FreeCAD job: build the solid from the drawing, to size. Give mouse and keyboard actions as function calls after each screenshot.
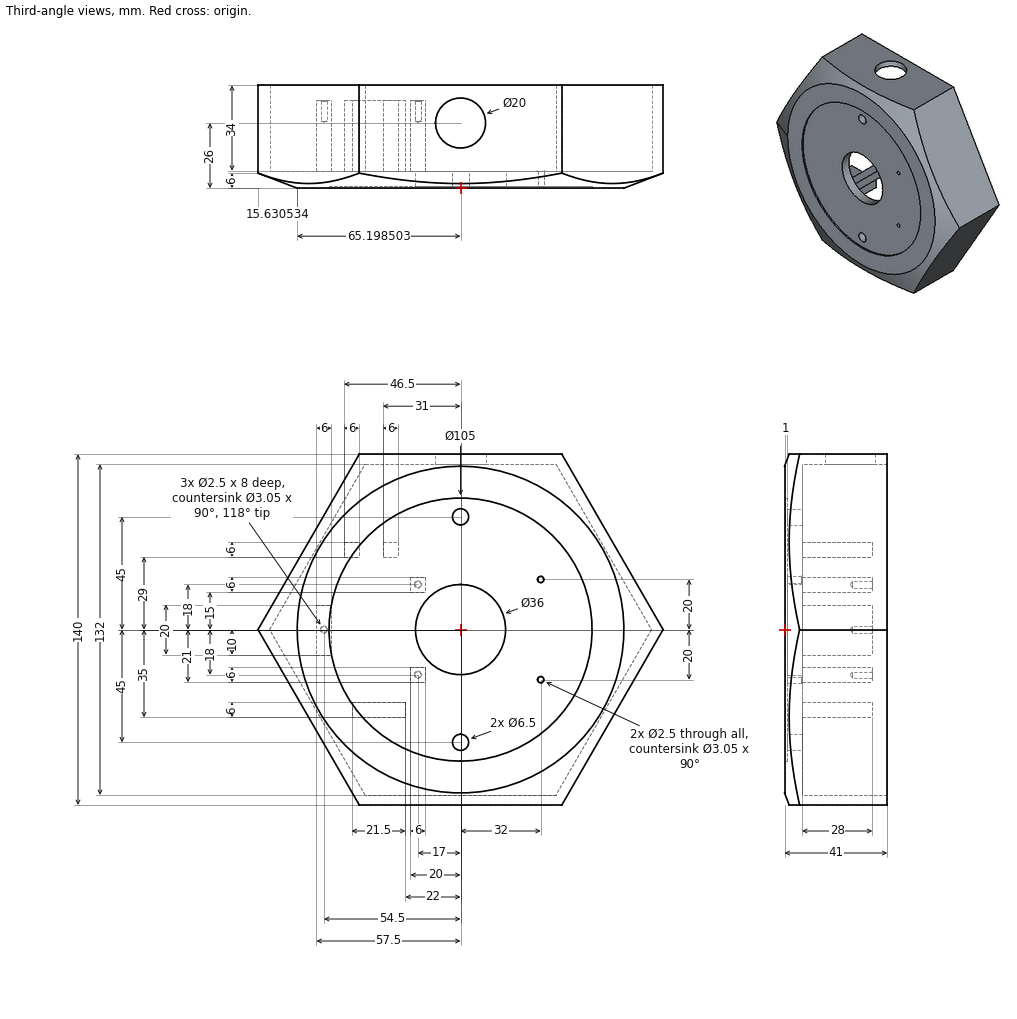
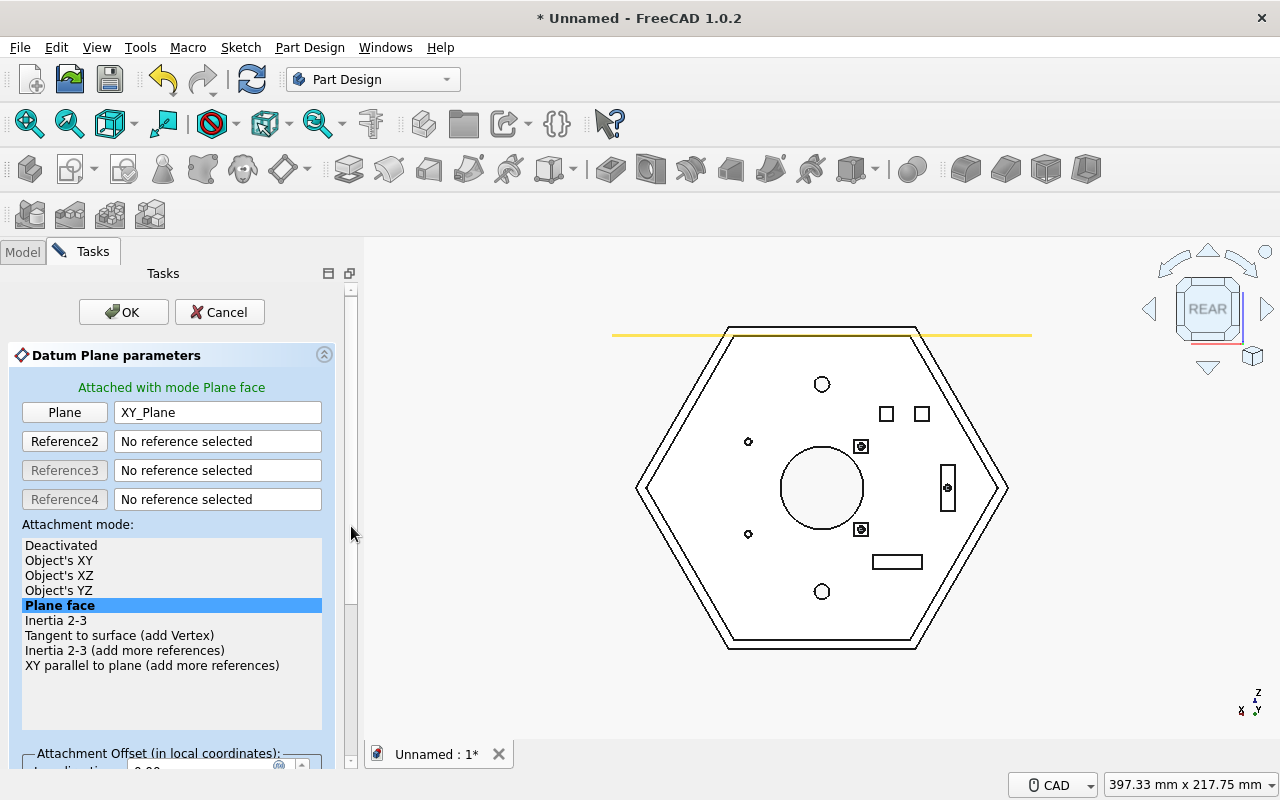
click(124, 312)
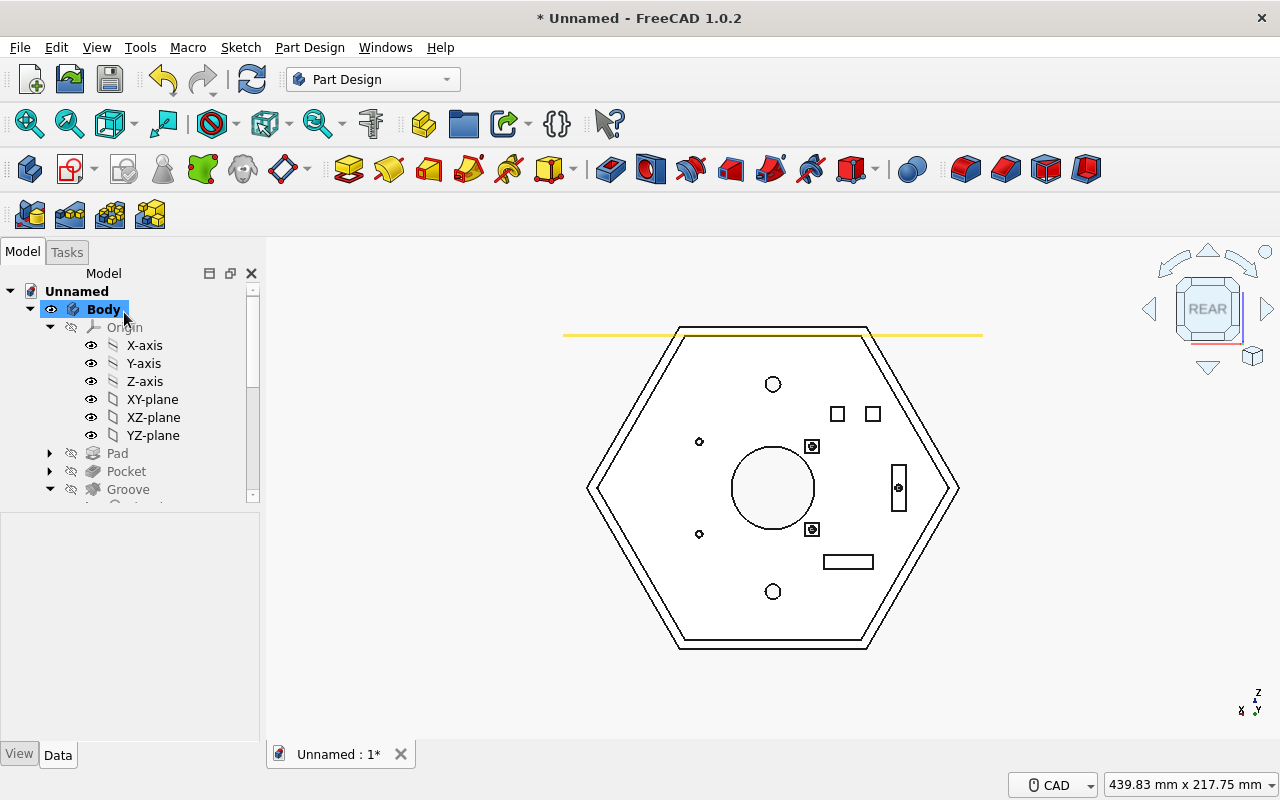
scroll(100, 395, down, 3)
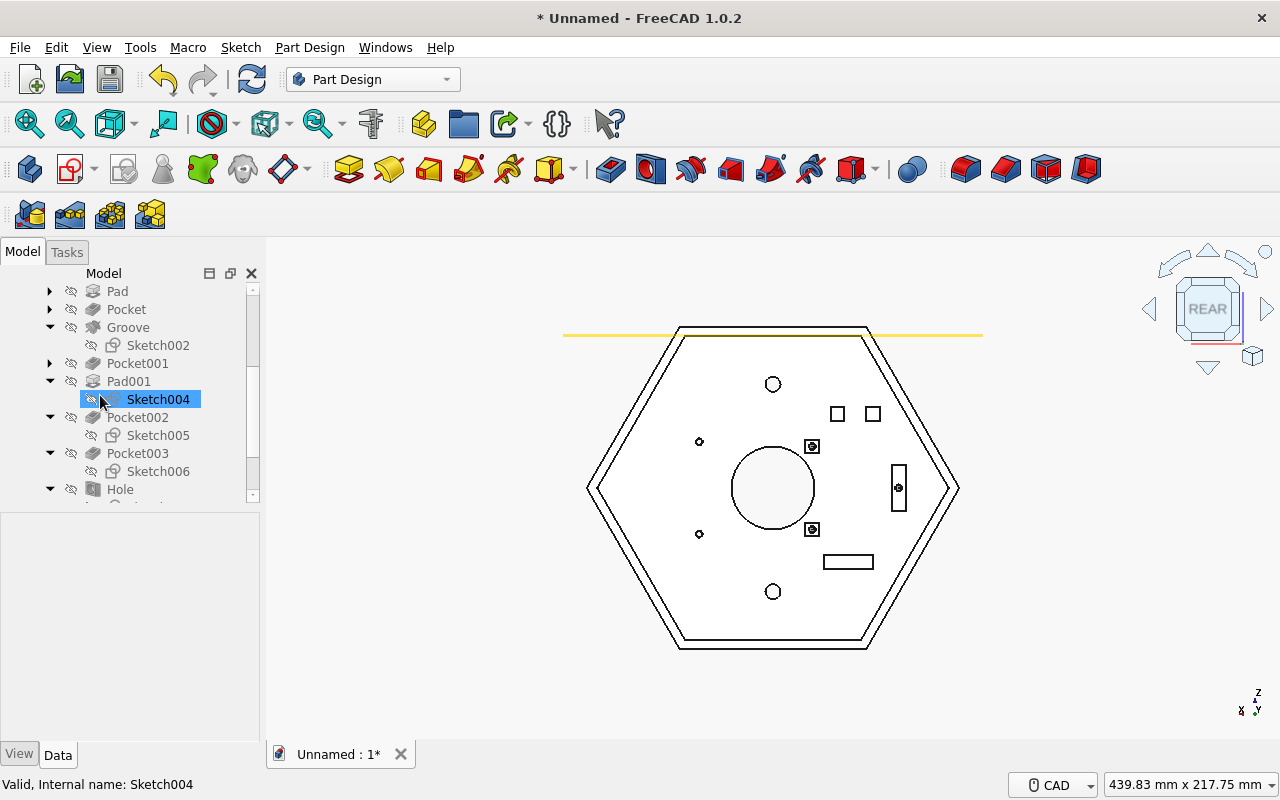
scroll(140, 395, up, 15)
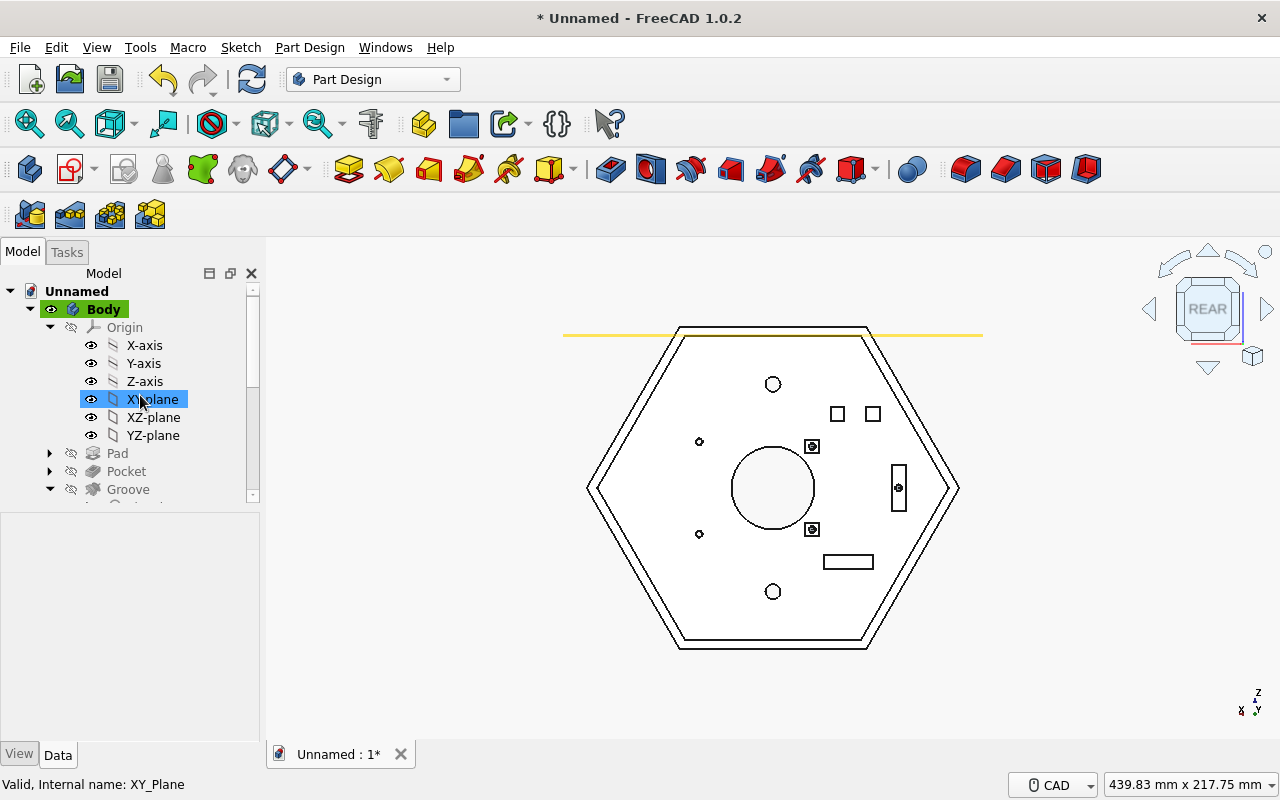
scroll(100, 395, down, 6)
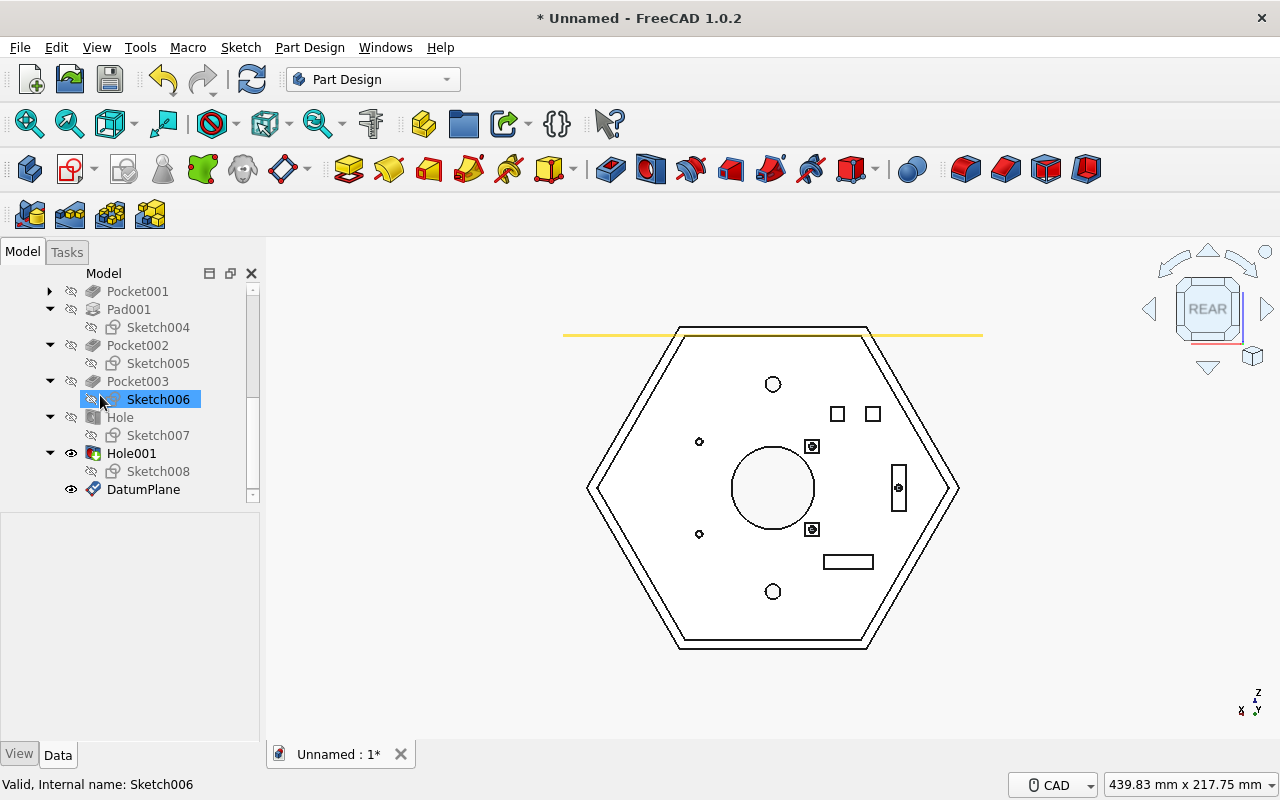
click(116, 489)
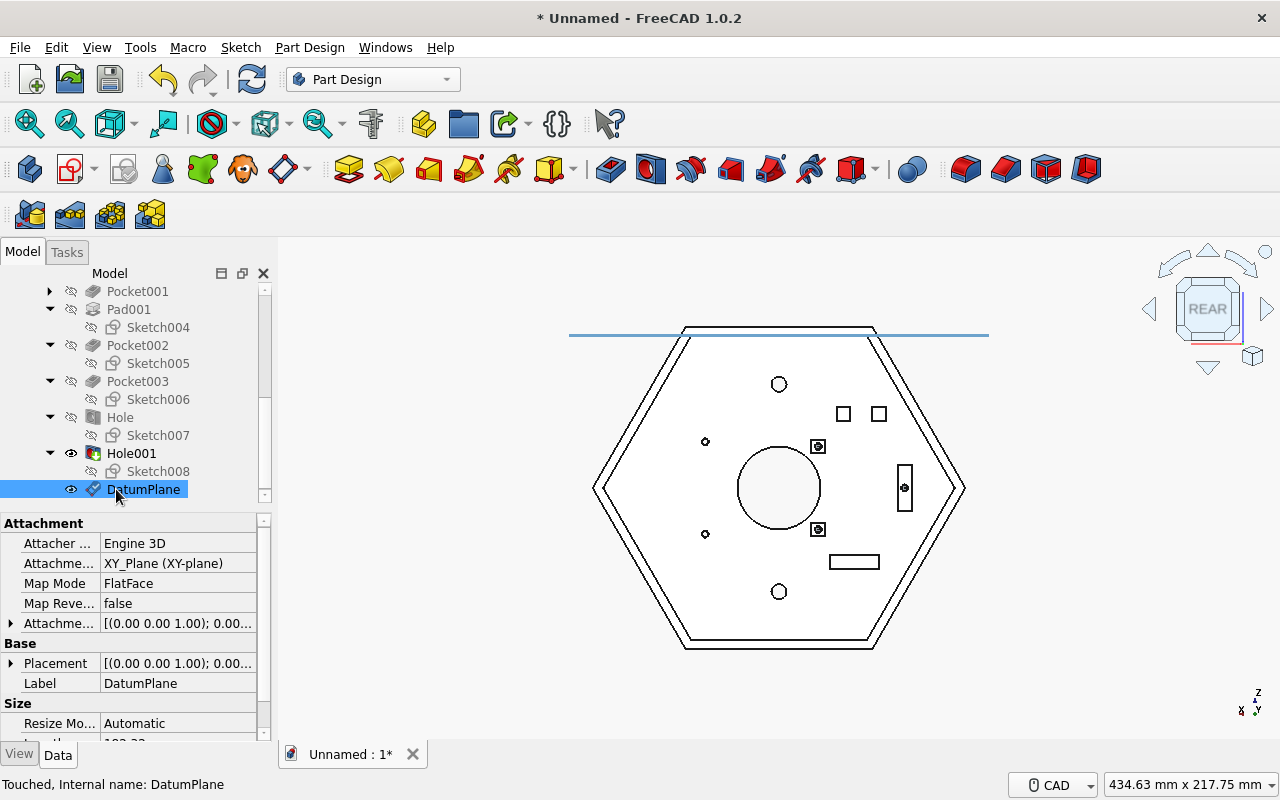
click(70, 170)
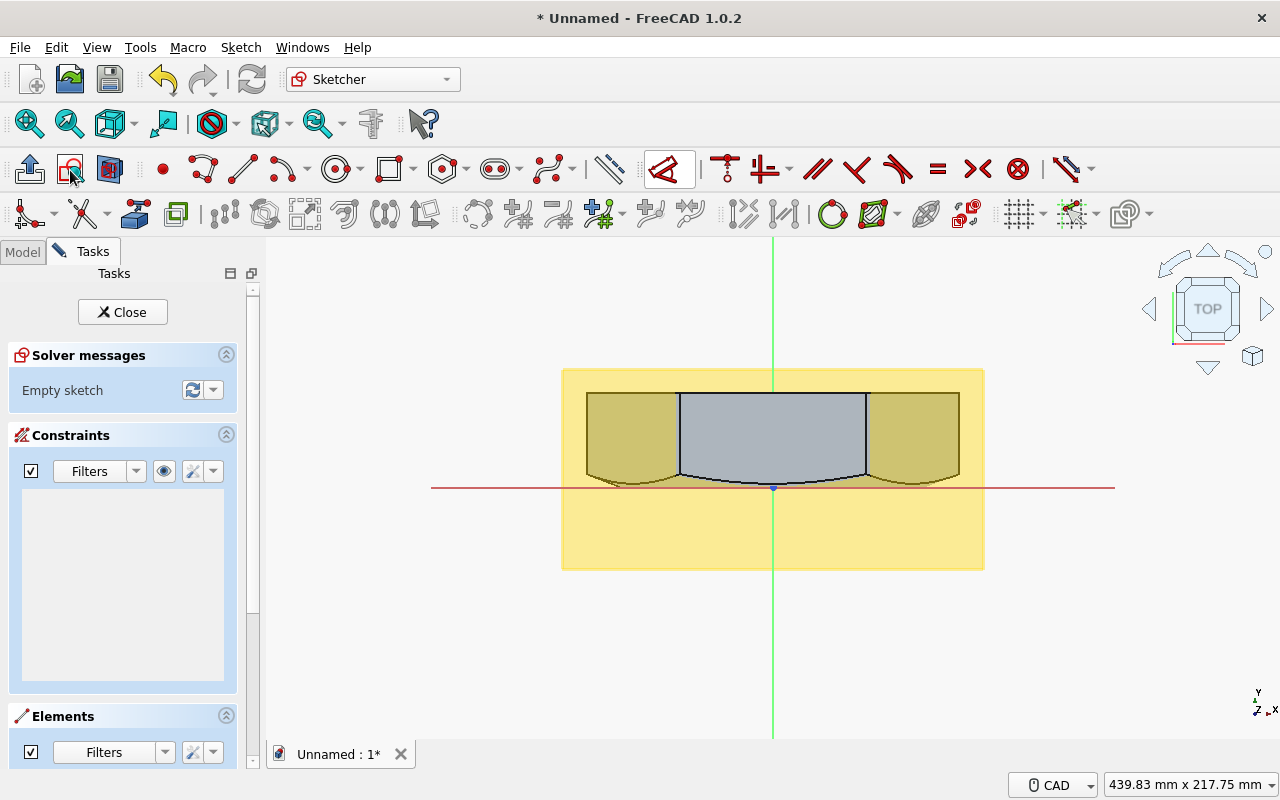
key(q)
key(s)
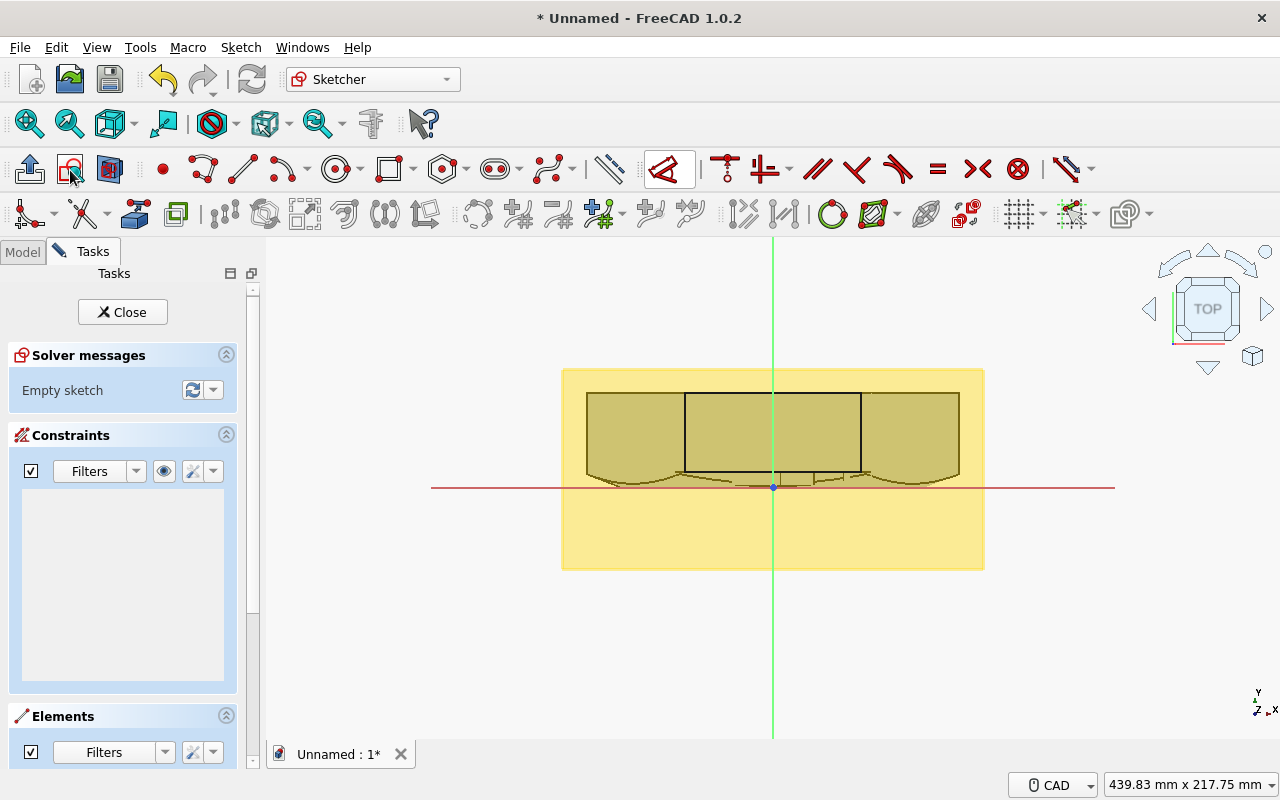
scroll(795, 433, up, 7)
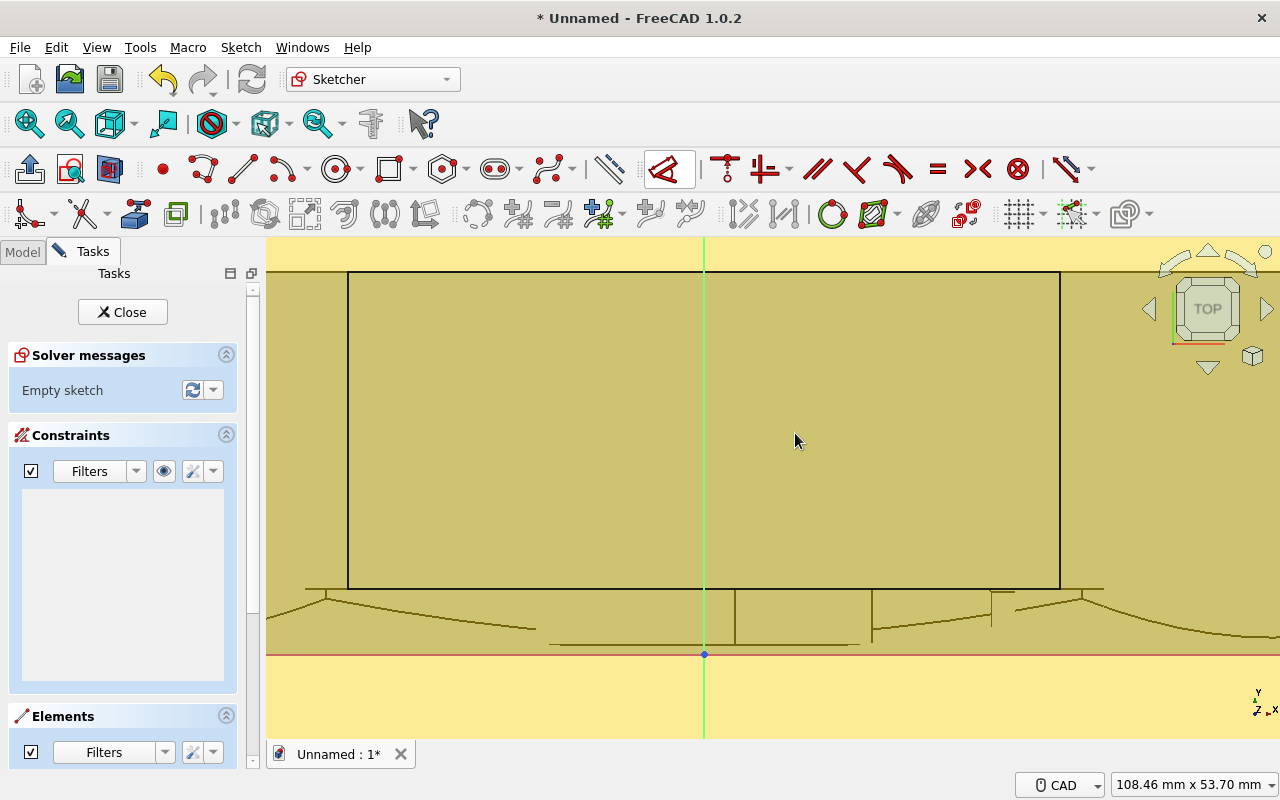
click(336, 170)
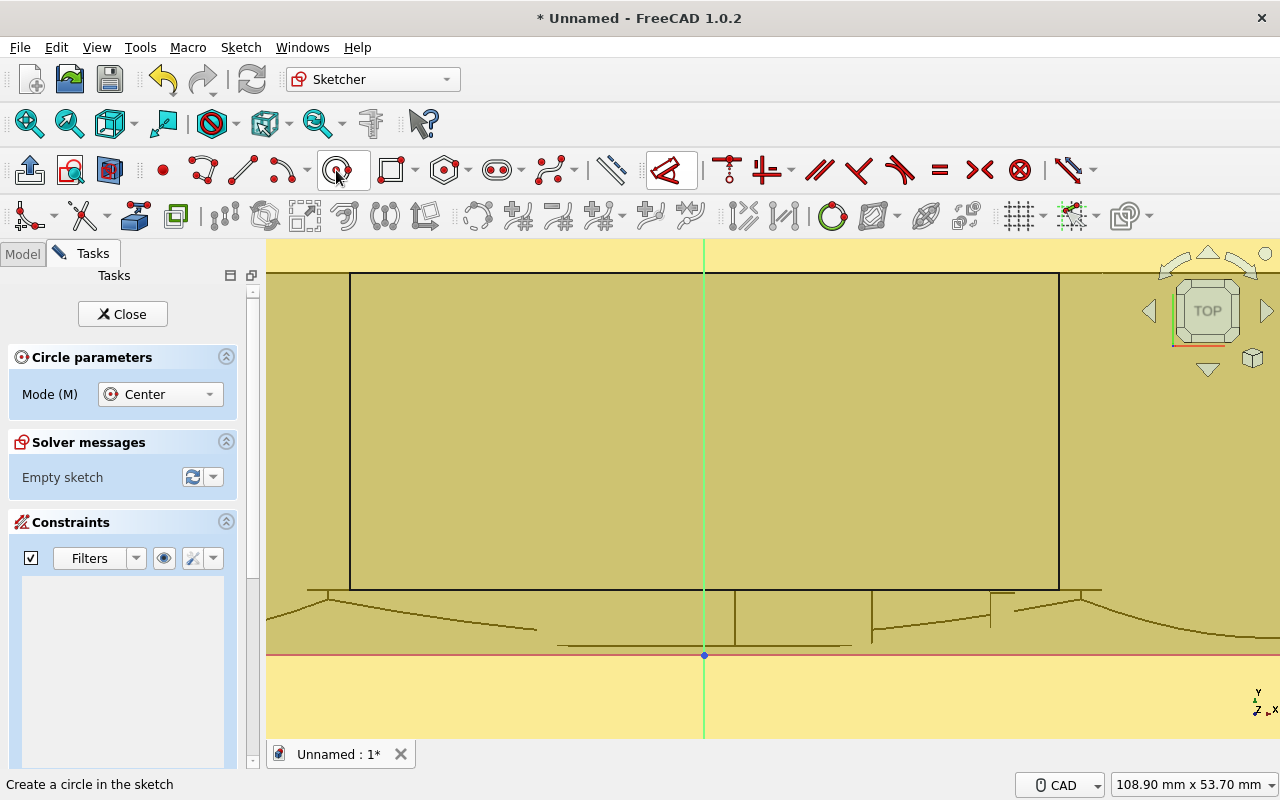
click(704, 413)
move(770, 347)